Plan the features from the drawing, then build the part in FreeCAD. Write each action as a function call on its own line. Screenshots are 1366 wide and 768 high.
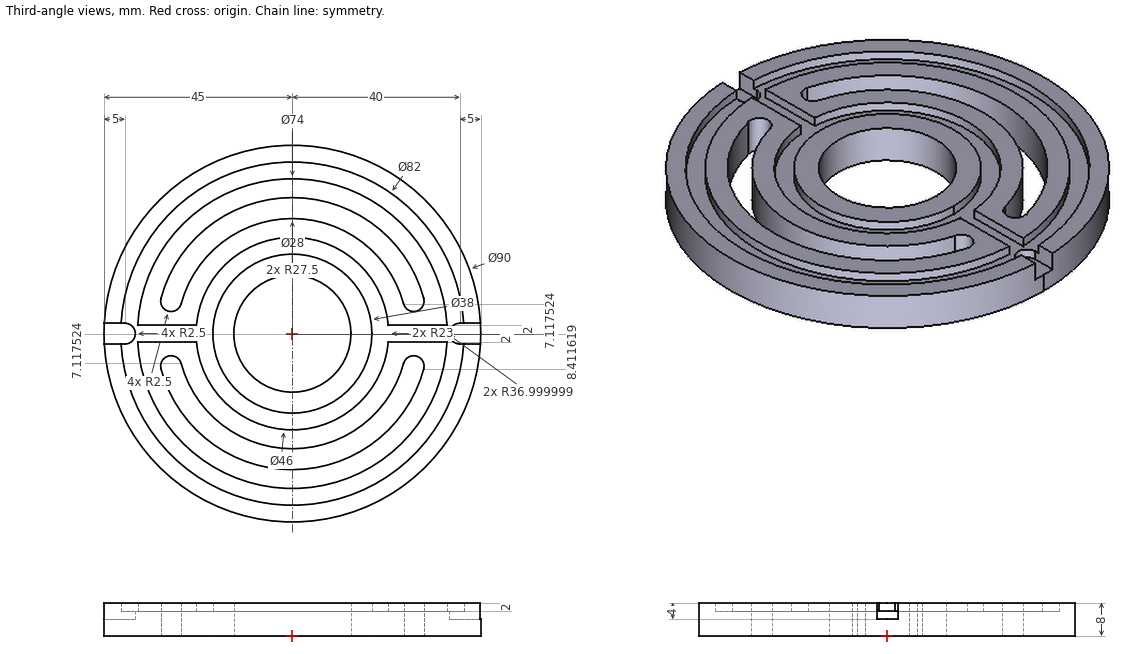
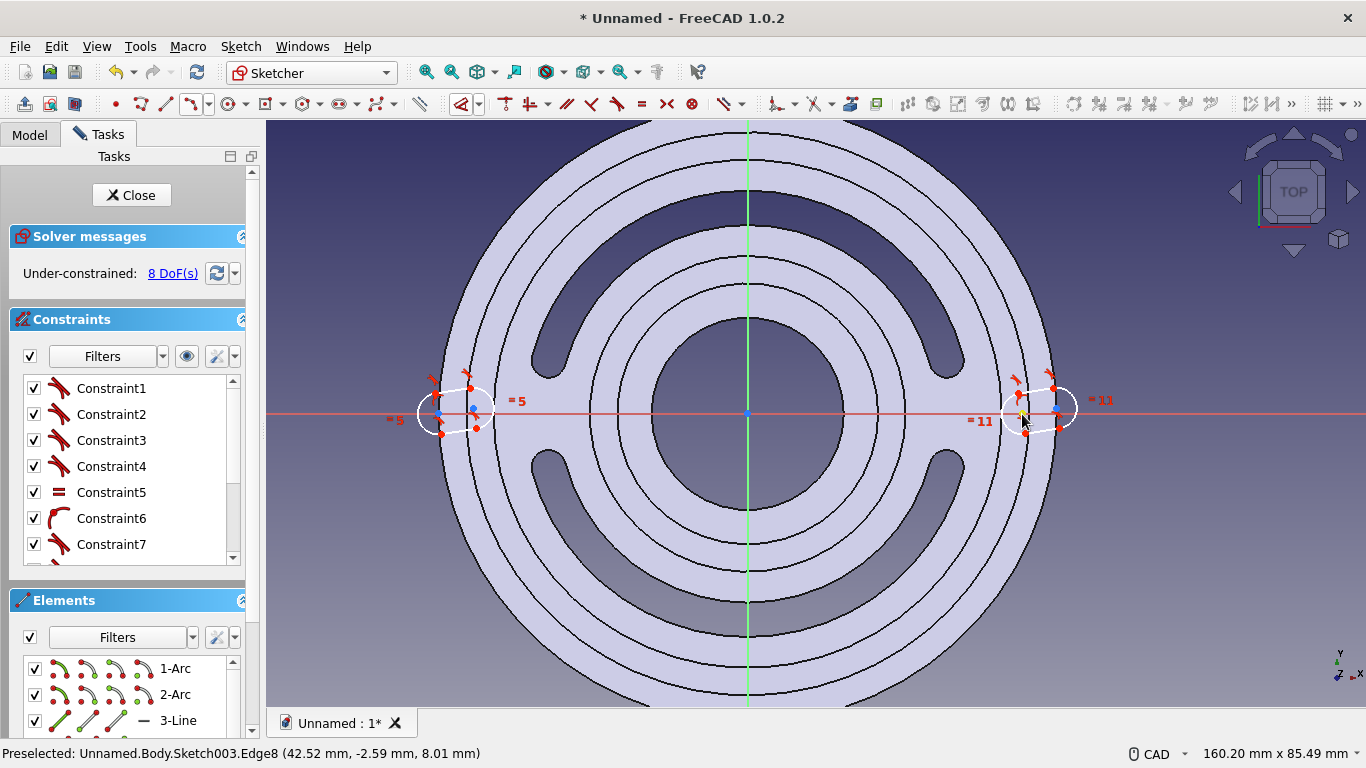
scroll(446, 392, up, 2)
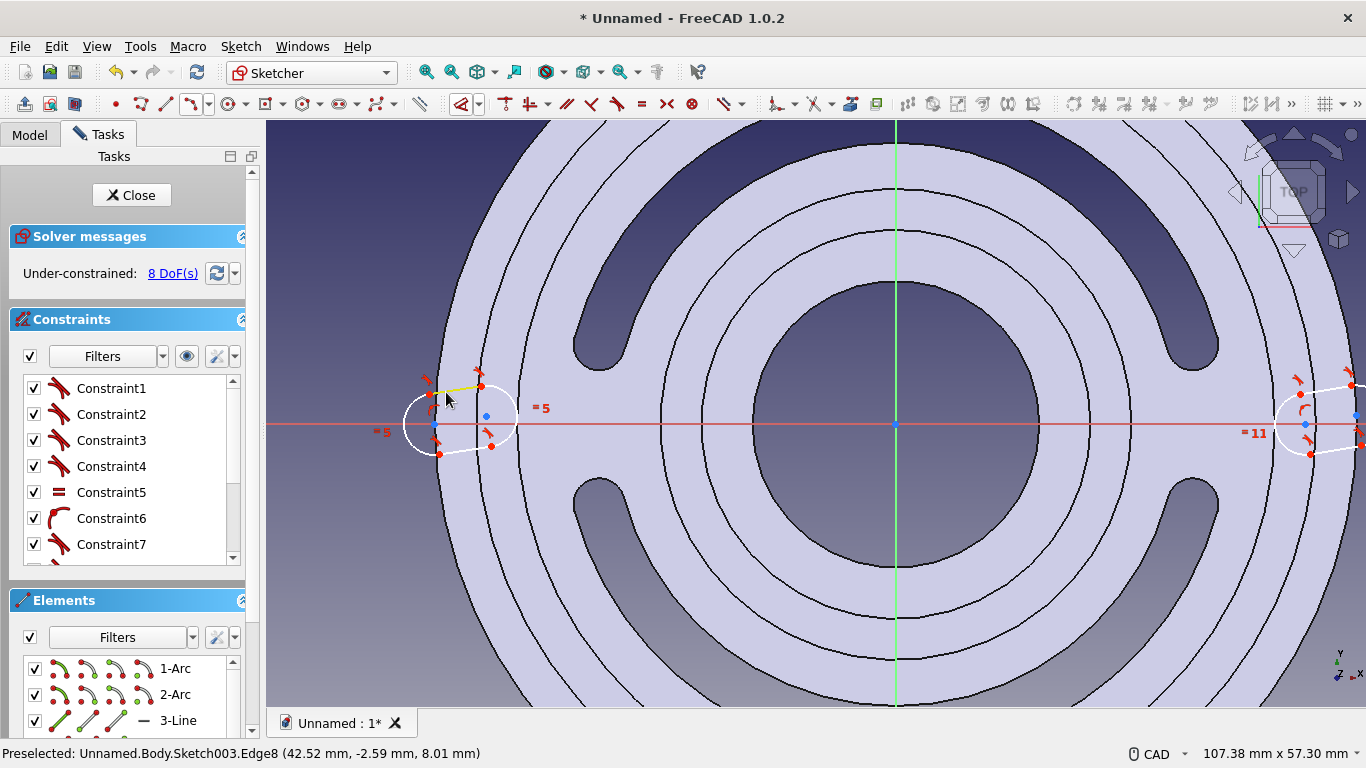
click(445, 392)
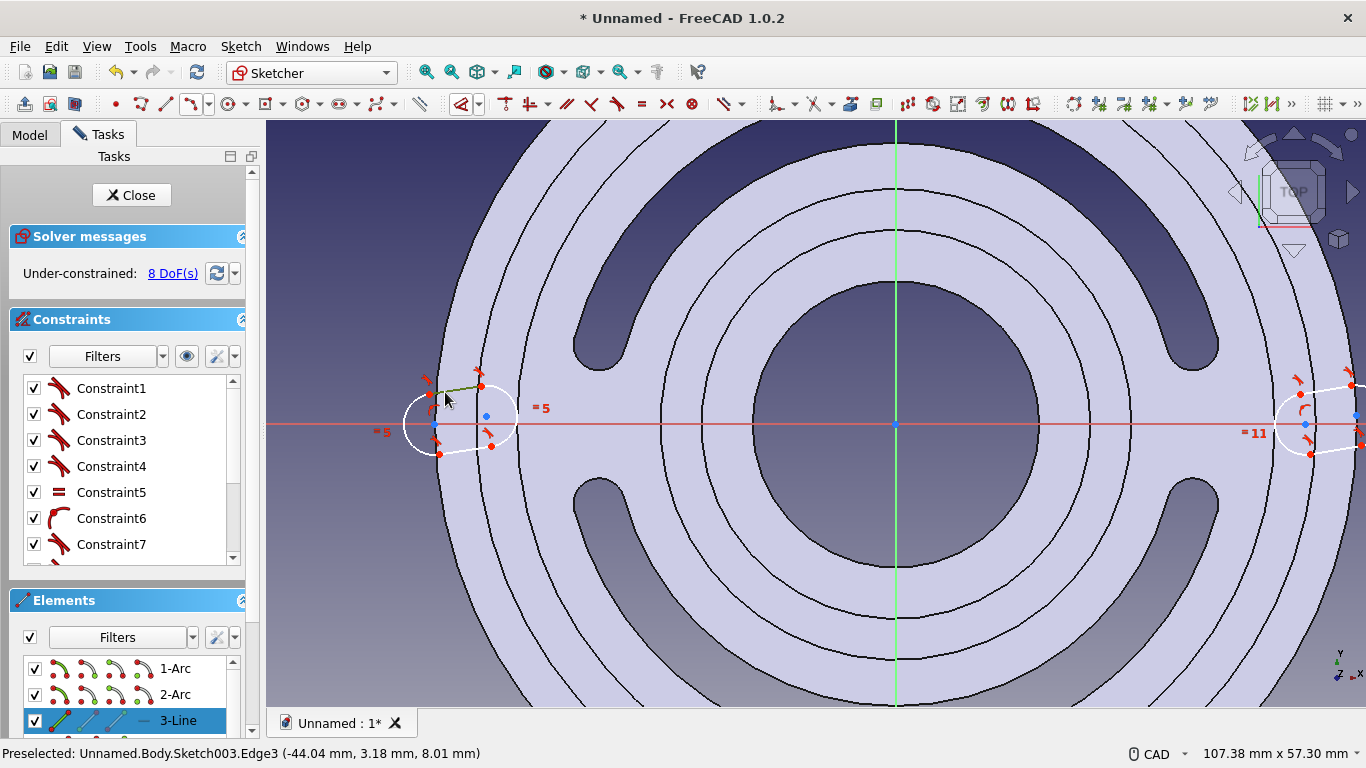
key(h)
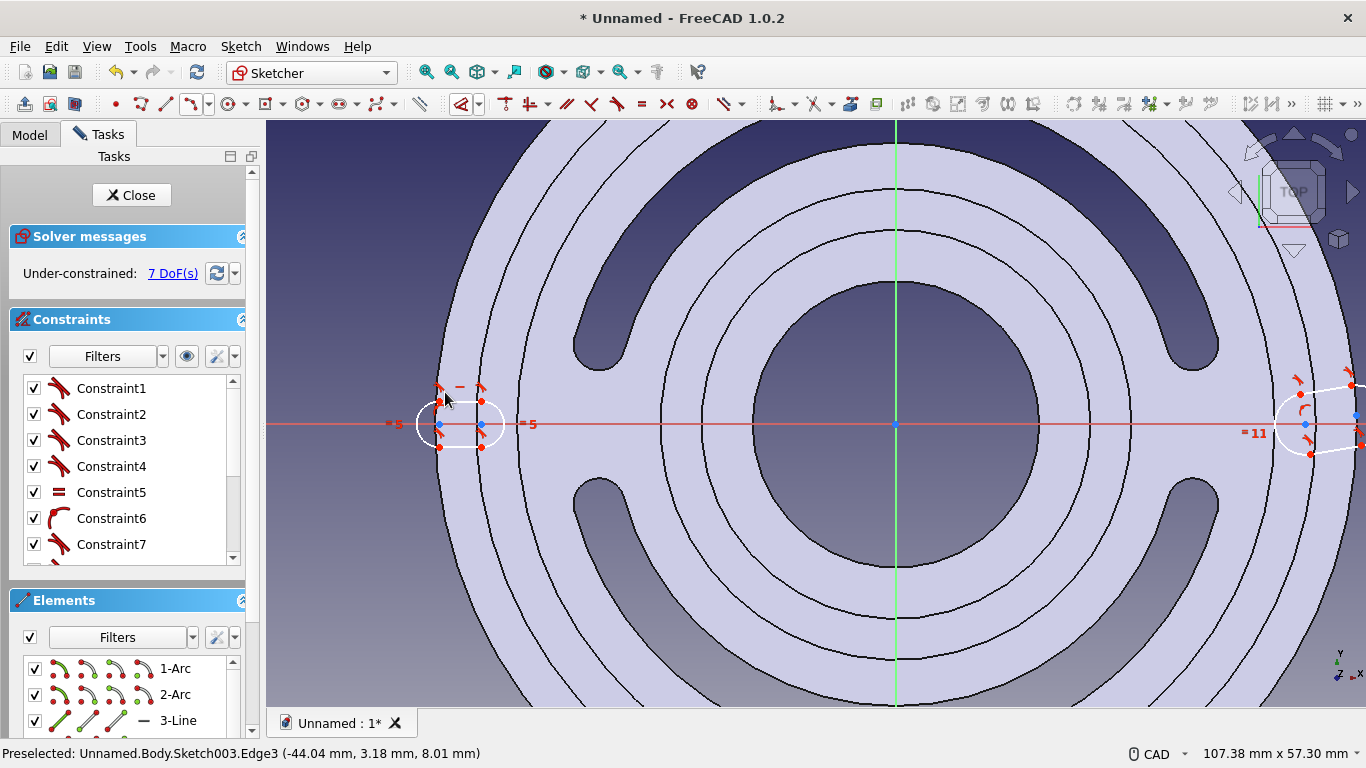
scroll(446, 391, down, 2)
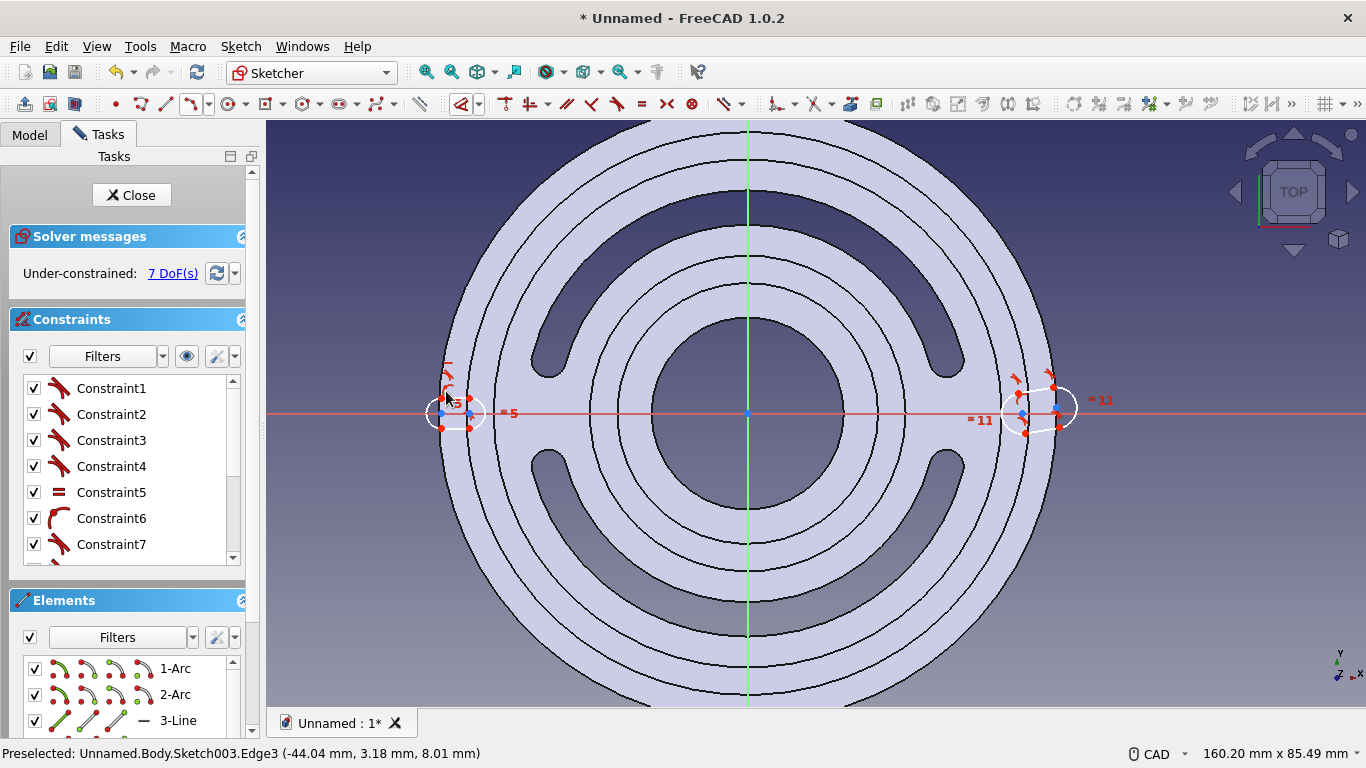
scroll(1029, 392, up, 2)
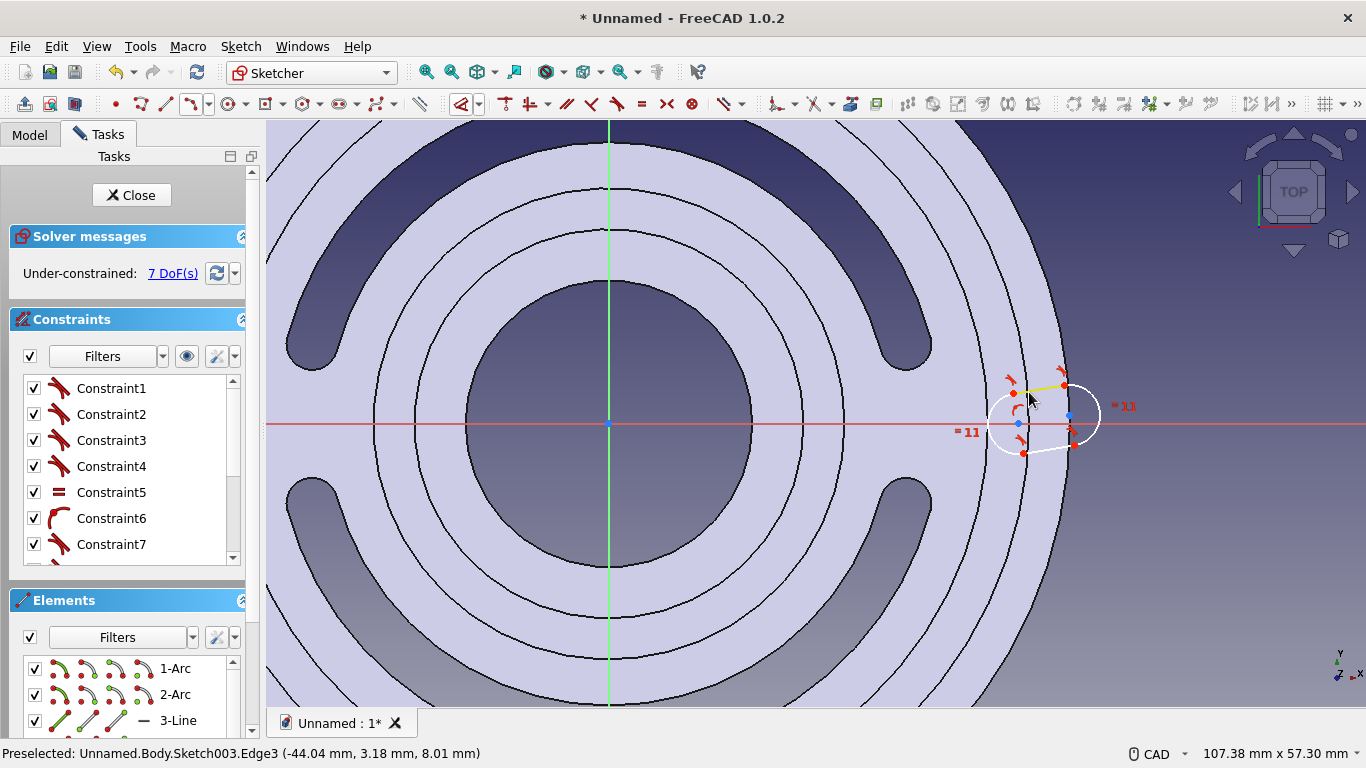
click(1029, 391)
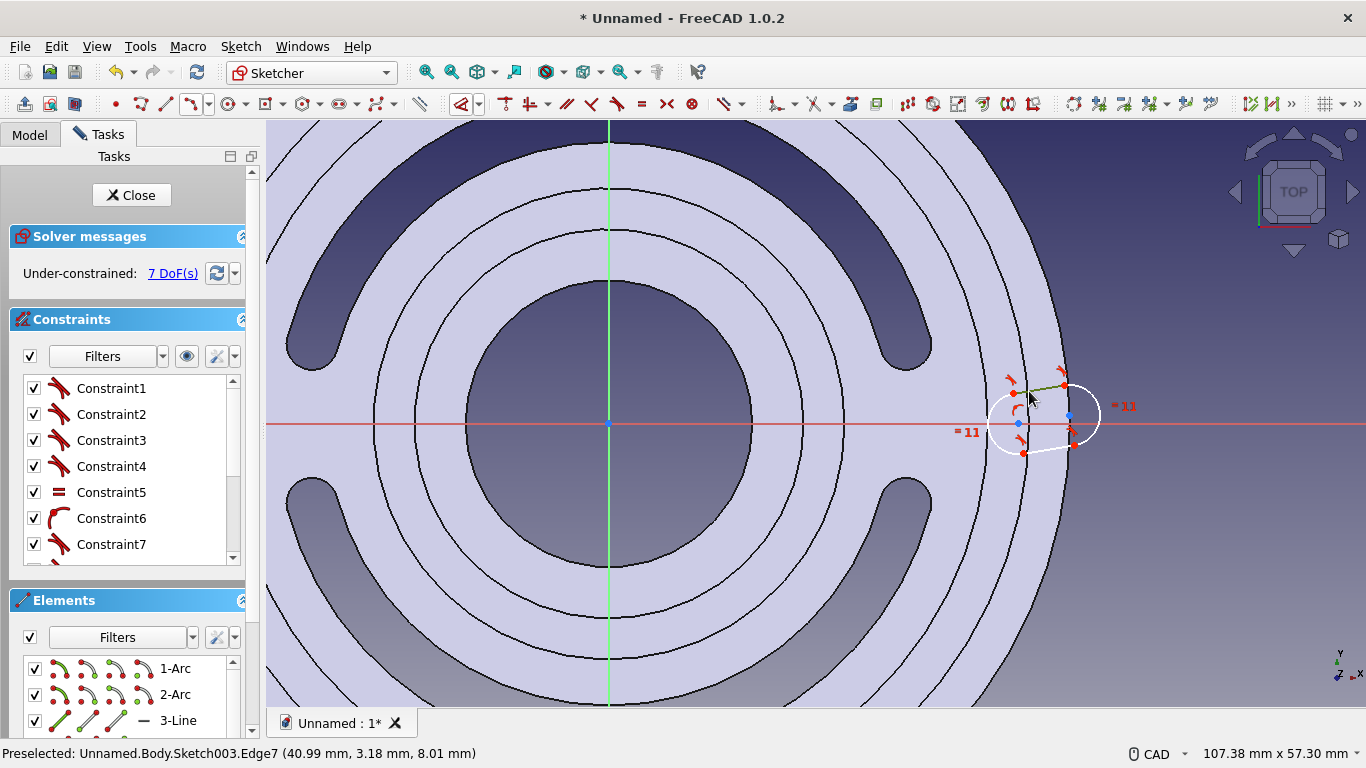
click(548, 104)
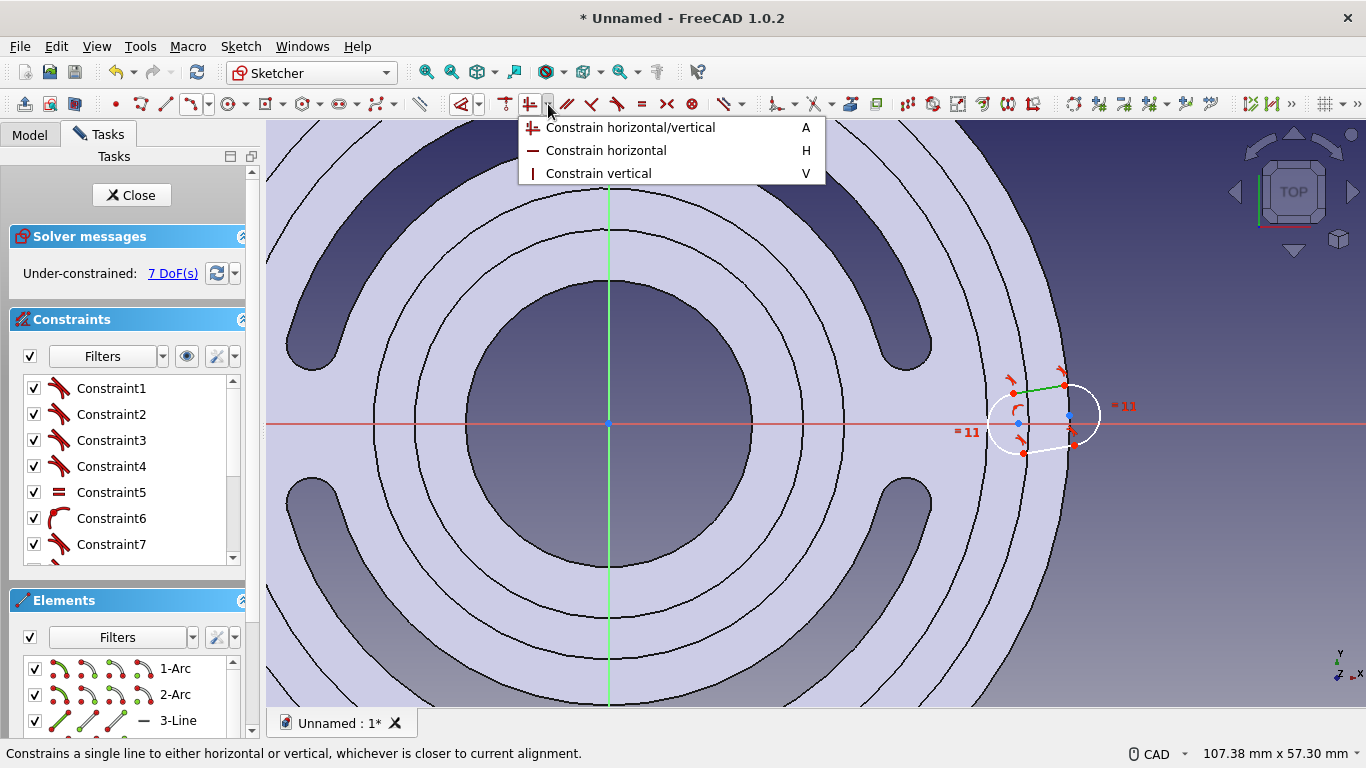
click(672, 150)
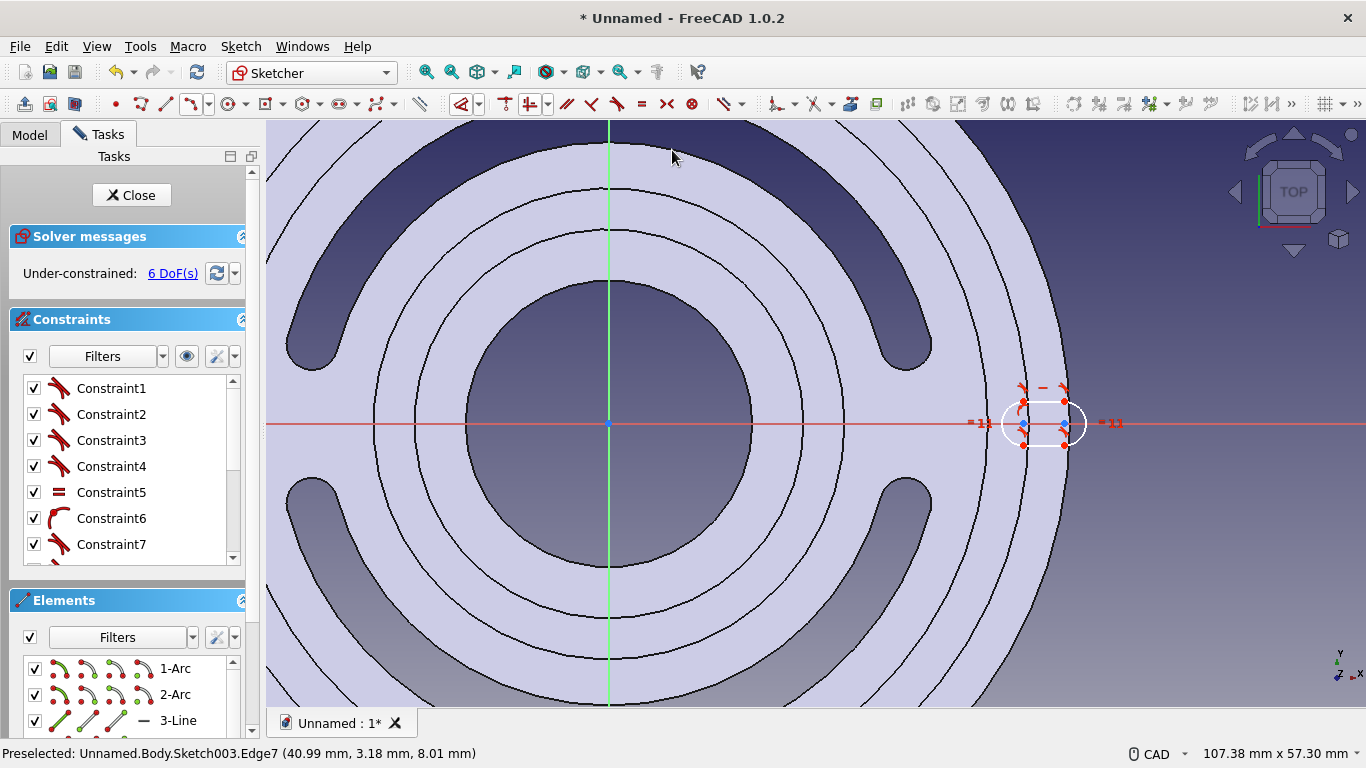
scroll(1029, 392, down, 2)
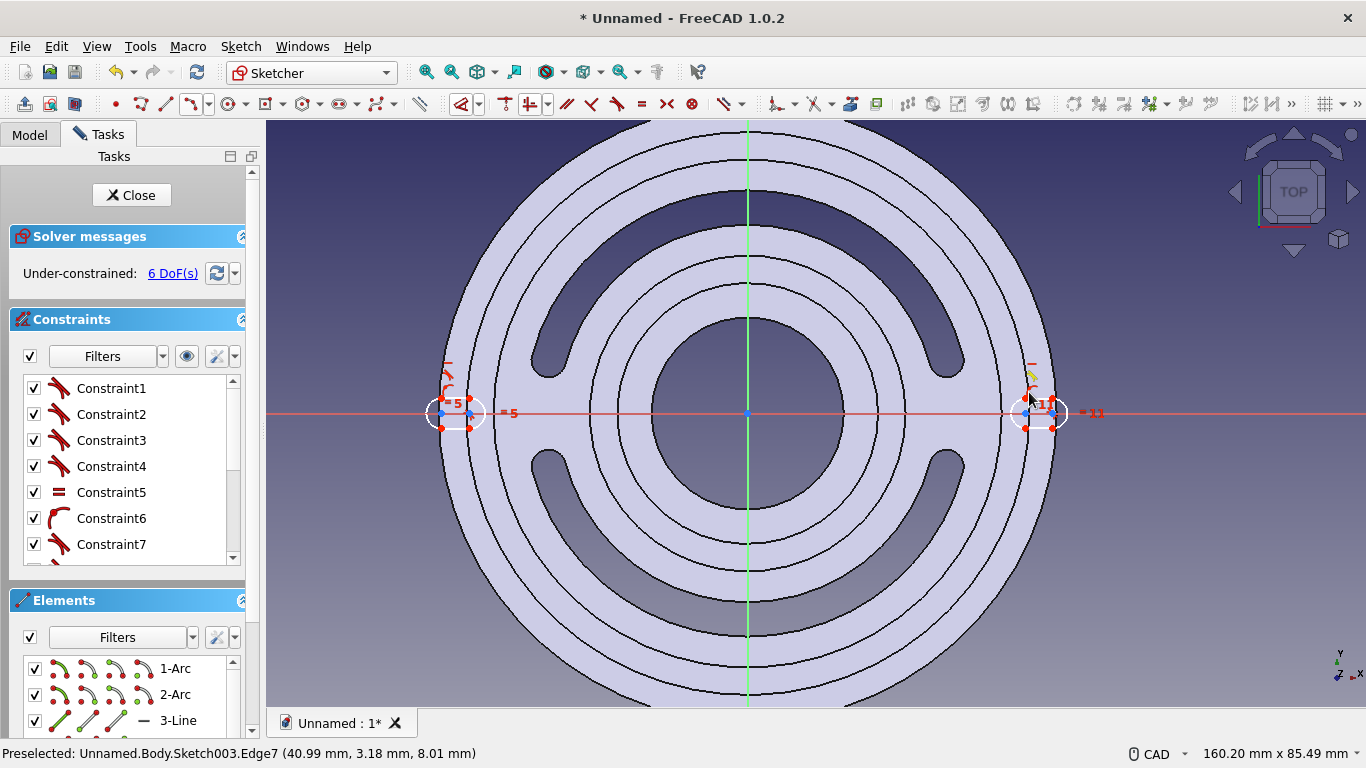
scroll(429, 405, up, 3)